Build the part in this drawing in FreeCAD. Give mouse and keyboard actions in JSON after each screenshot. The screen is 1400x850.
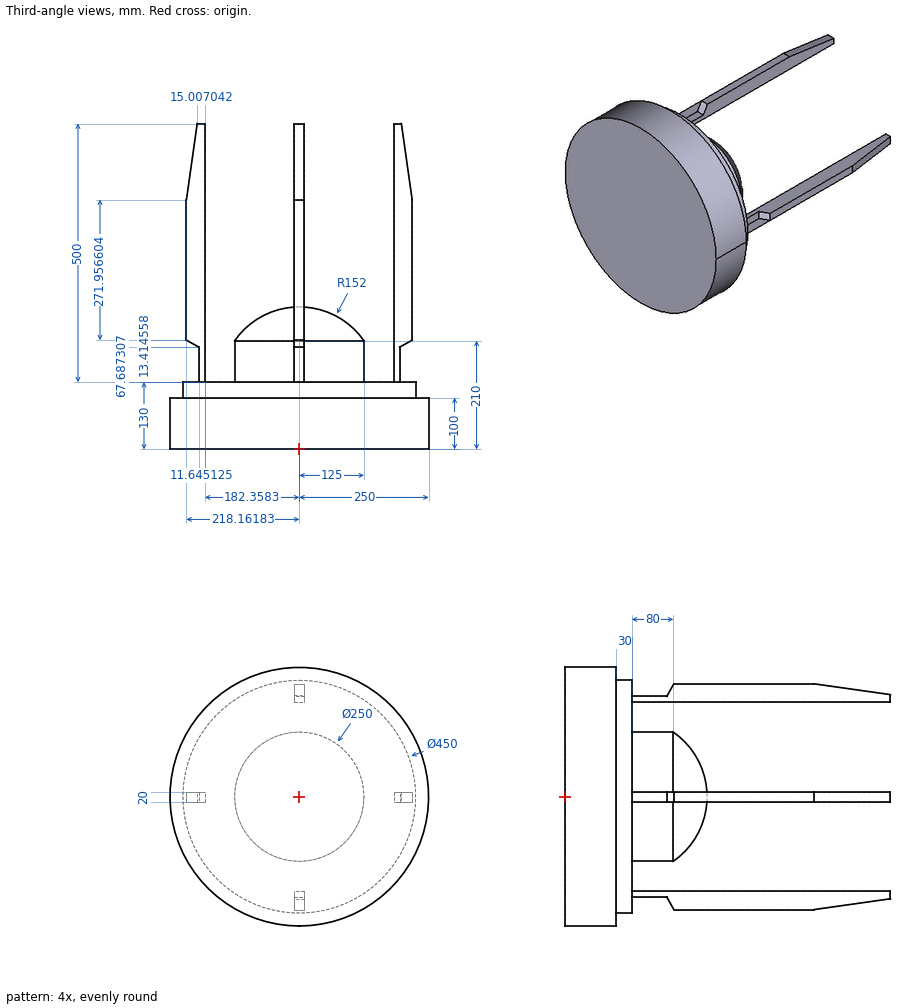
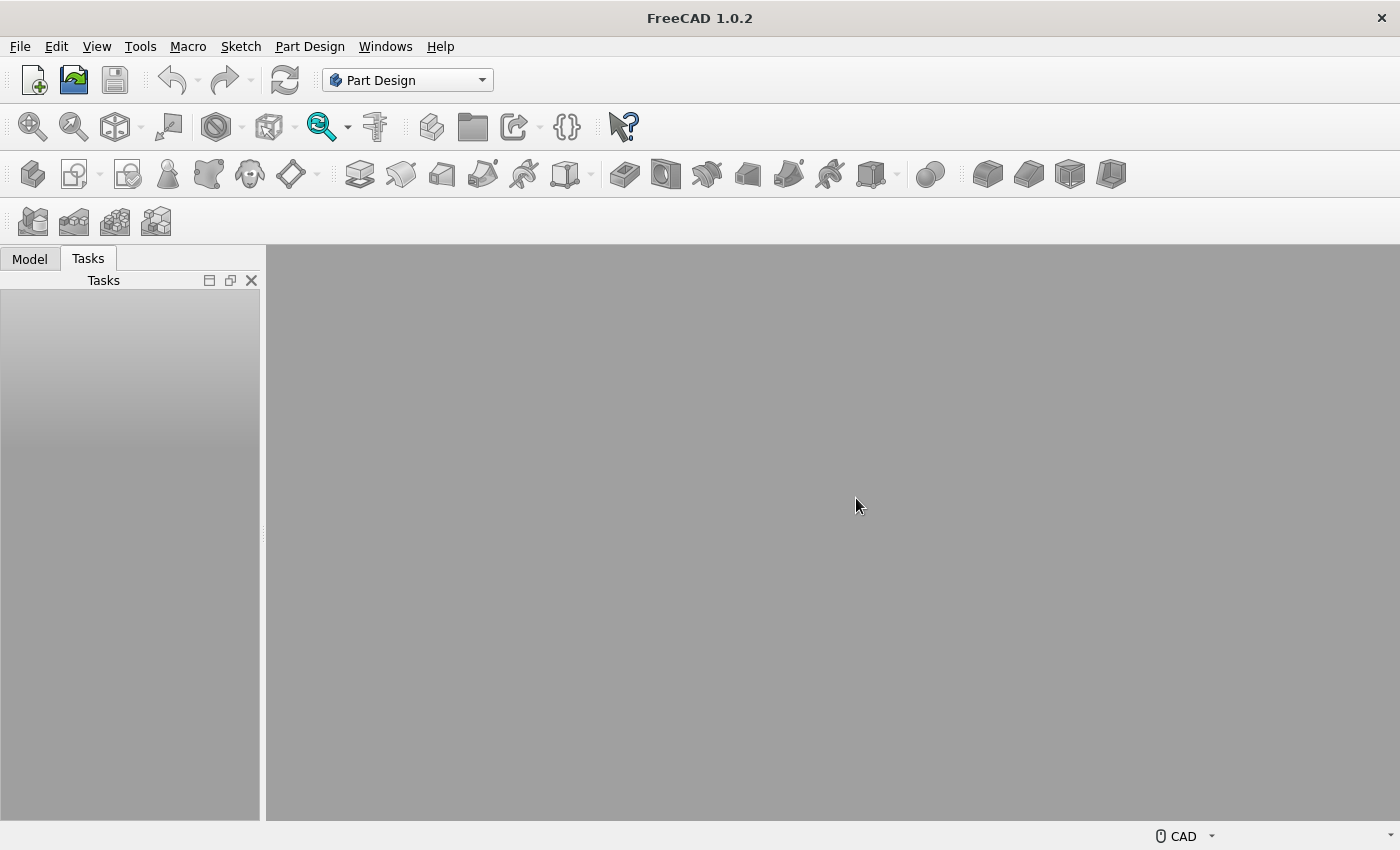
{"action": "left_click", "coordinate": [33, 80]}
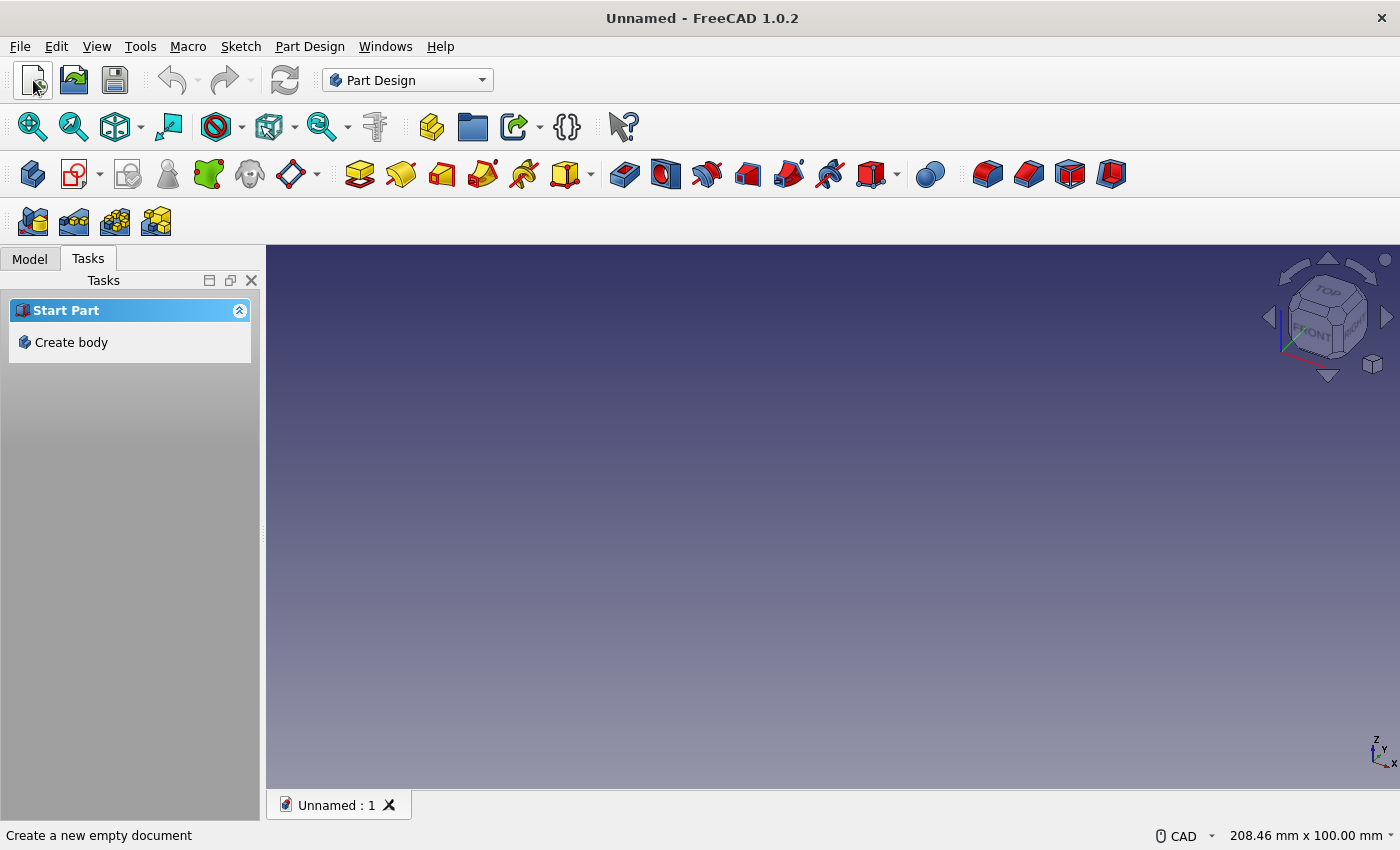
{"action": "left_click", "coordinate": [74, 174]}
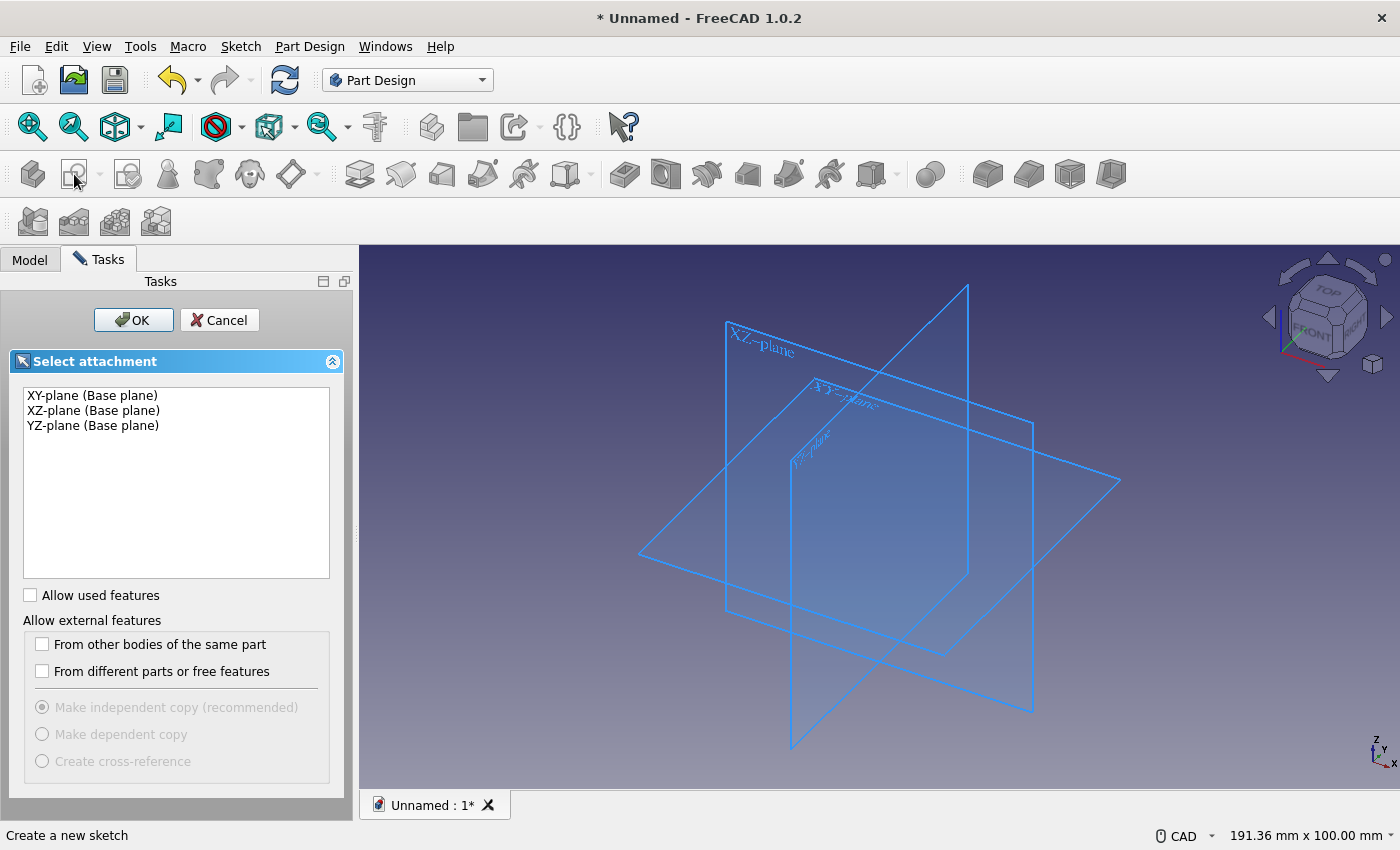
{"action": "left_click", "coordinate": [84, 396]}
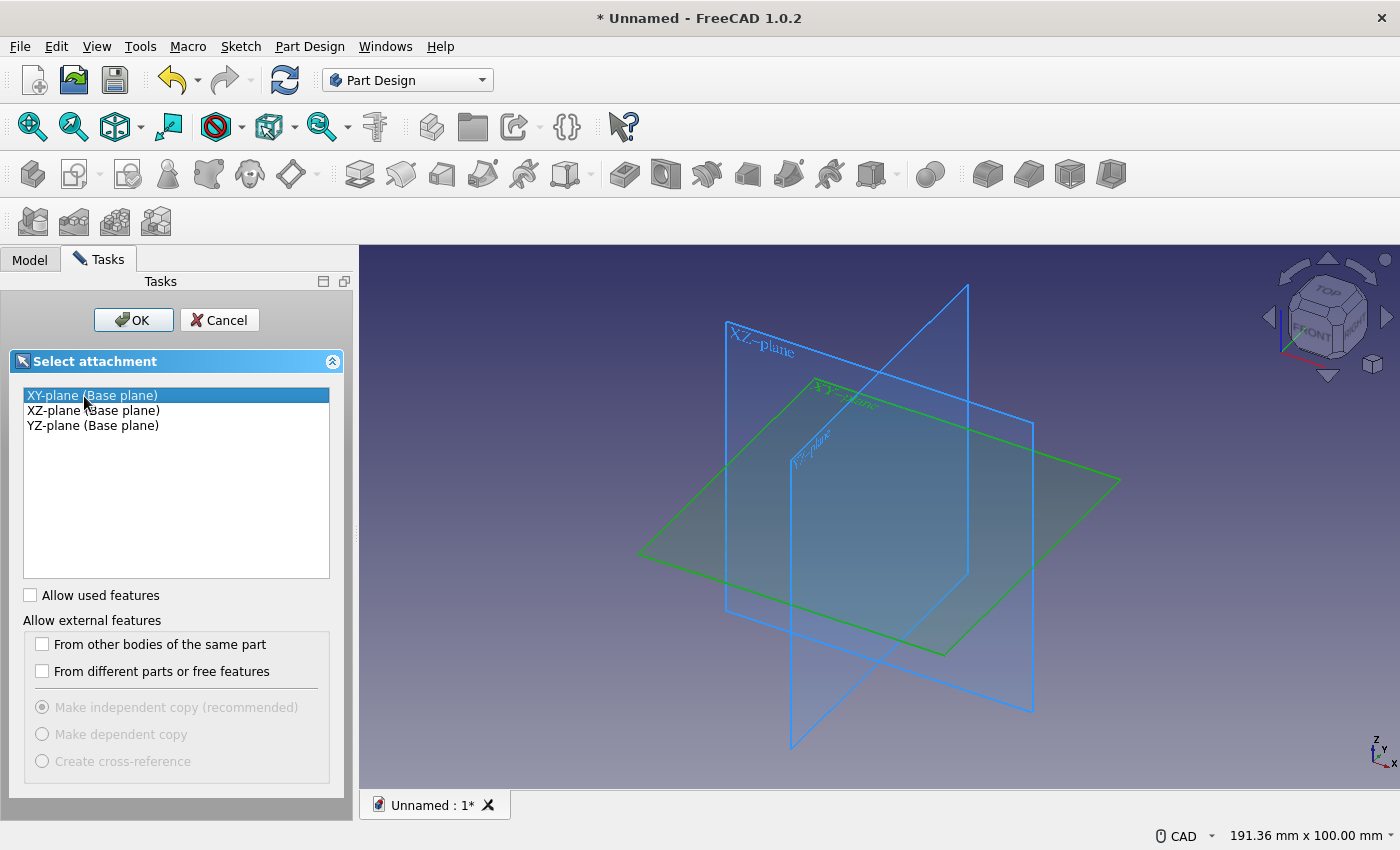
{"action": "left_click", "coordinate": [134, 320]}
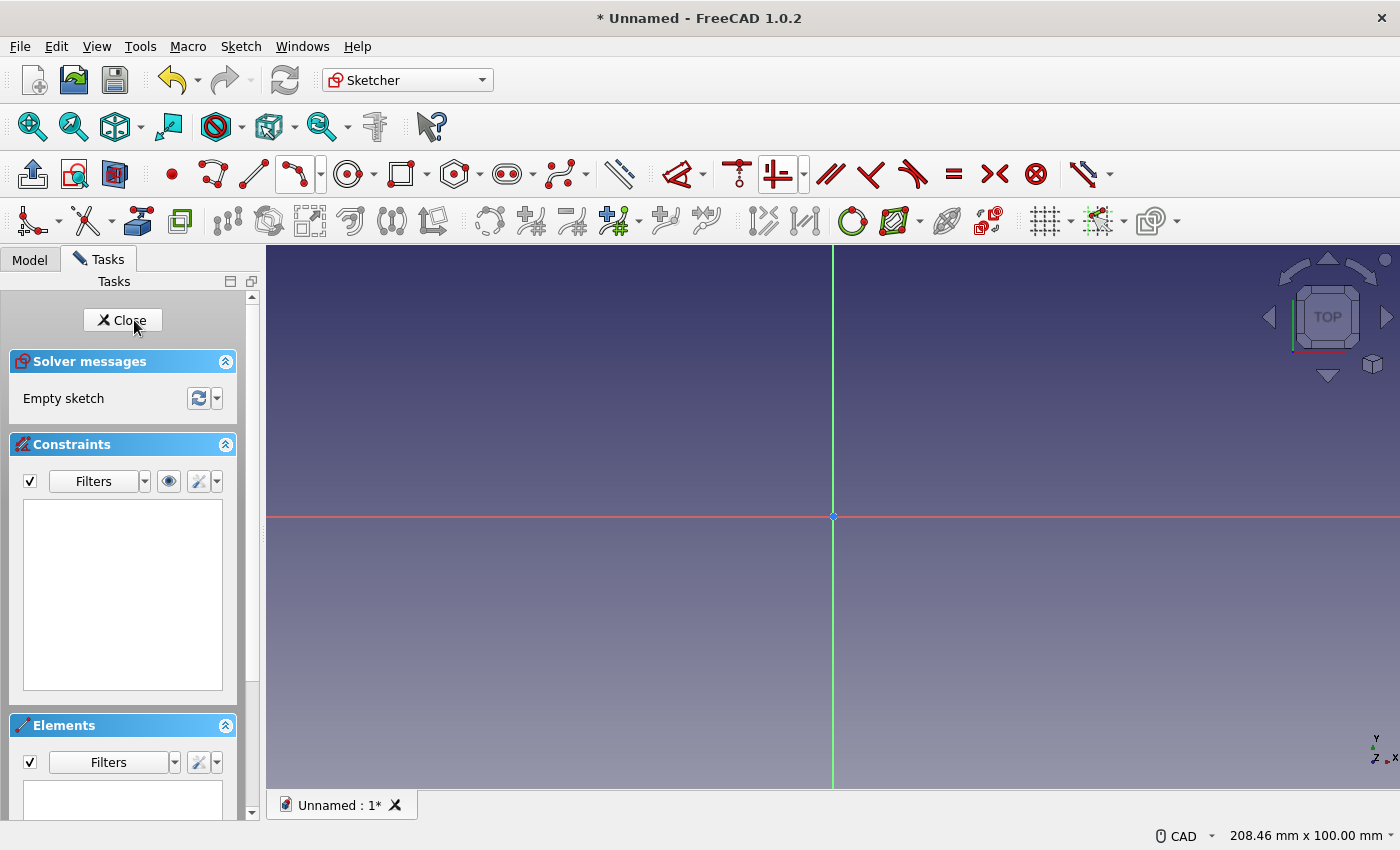
{"action": "scroll", "coordinate": [294, 739], "scroll_direction": "down", "scroll_amount": 4}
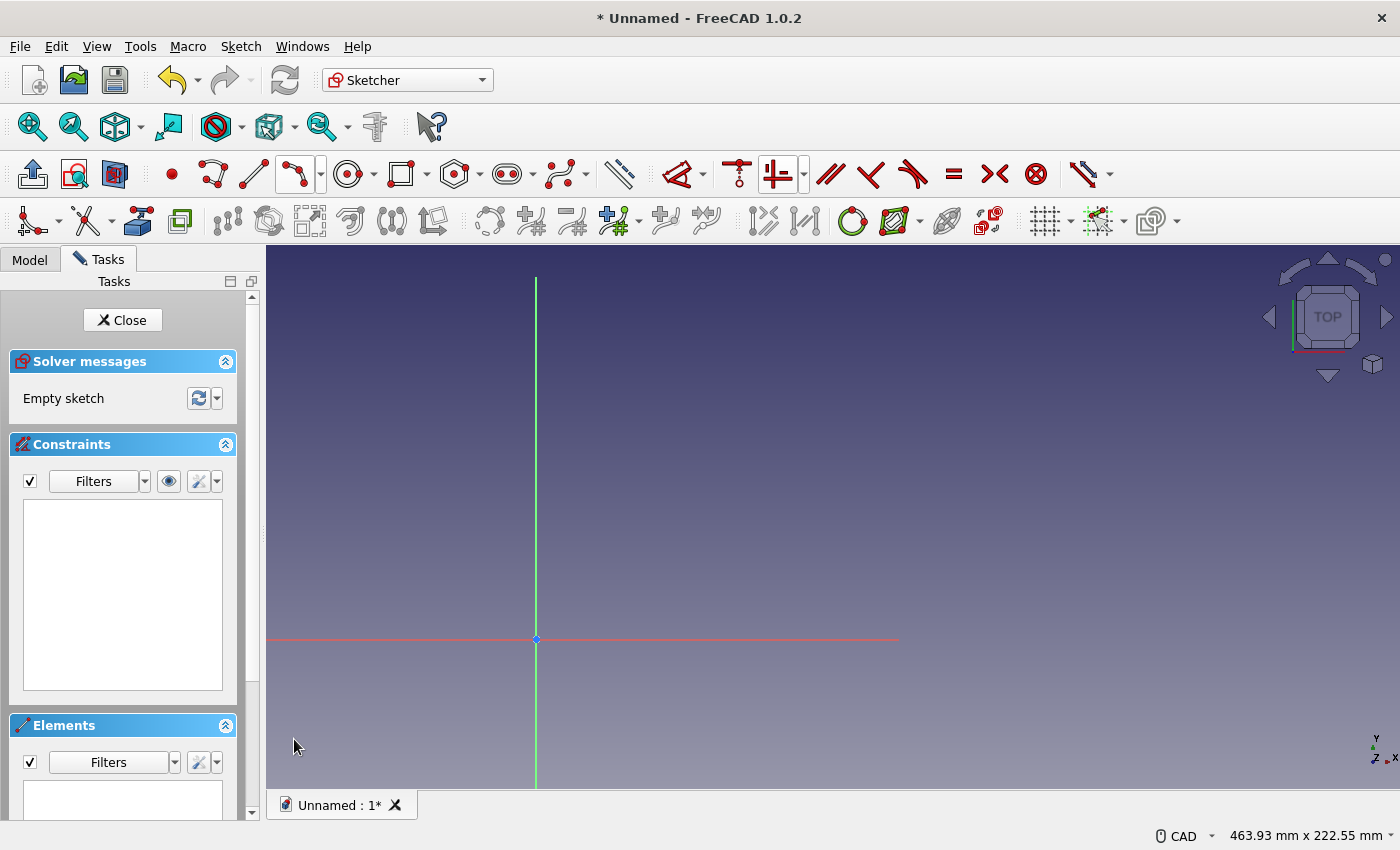
{"action": "left_click", "coordinate": [400, 174]}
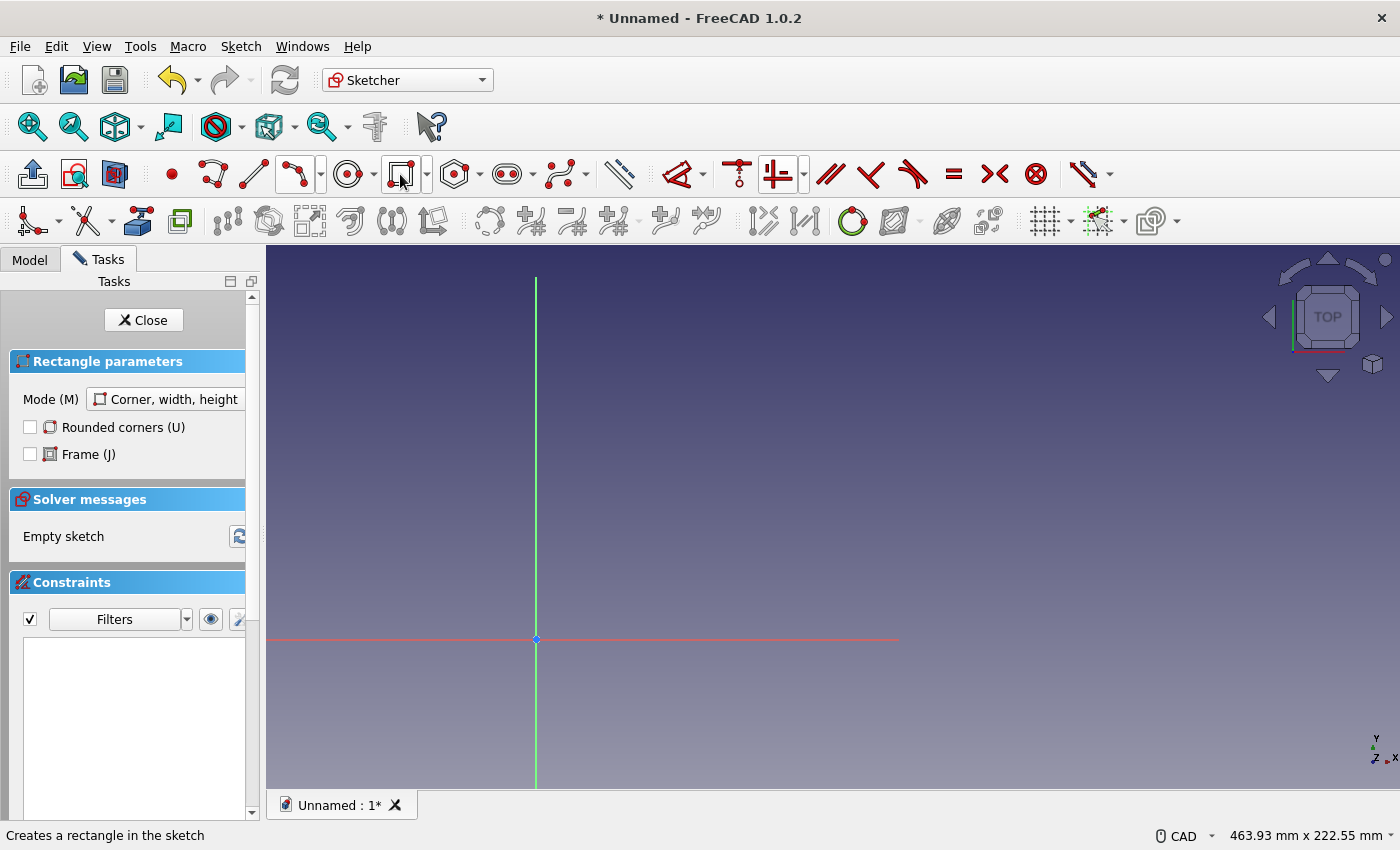
{"action": "left_click", "coordinate": [536, 640]}
{"action": "left_click", "coordinate": [1147, 395]}
{"action": "key", "text": "Escape"}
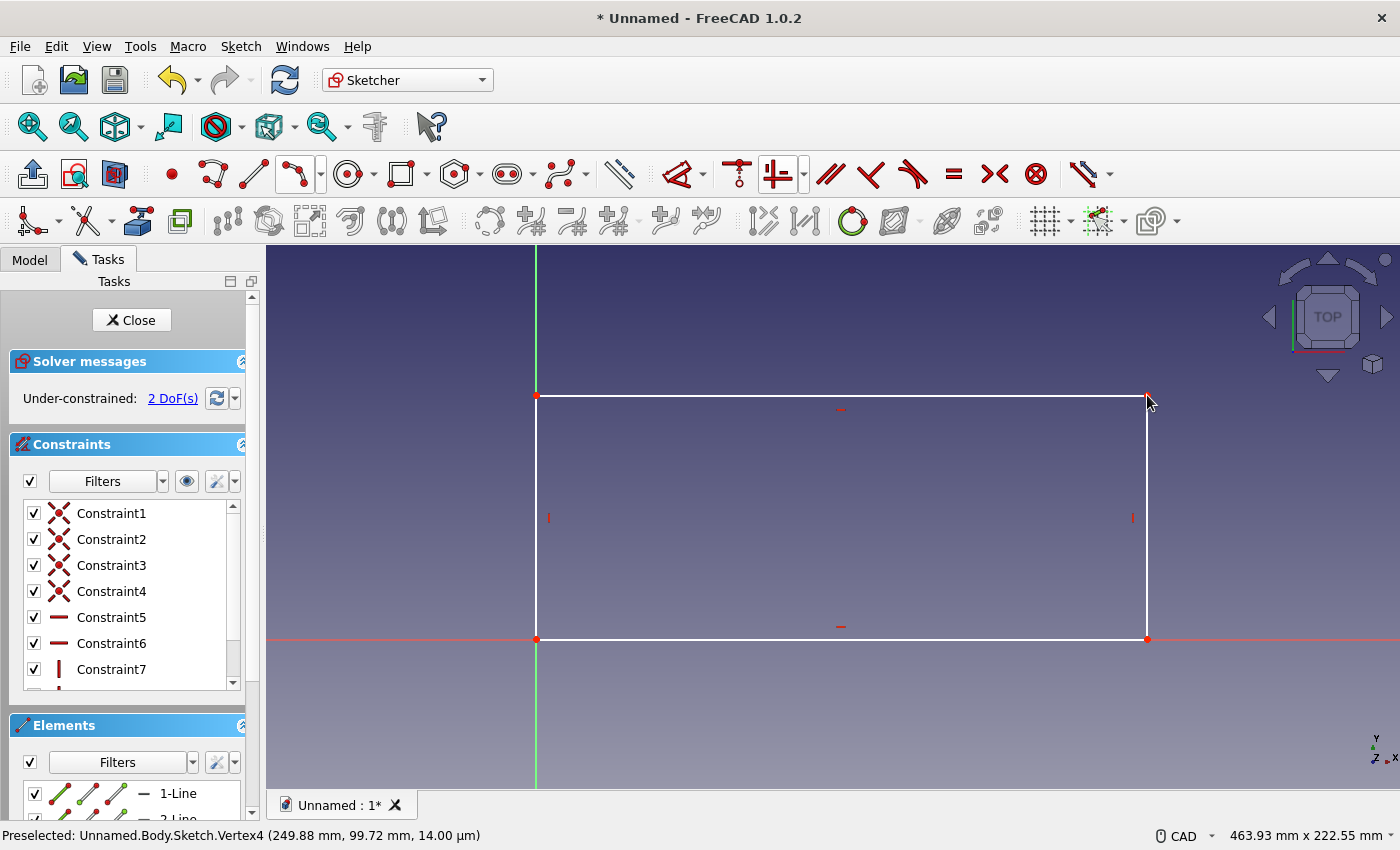
{"action": "left_click", "coordinate": [719, 640]}